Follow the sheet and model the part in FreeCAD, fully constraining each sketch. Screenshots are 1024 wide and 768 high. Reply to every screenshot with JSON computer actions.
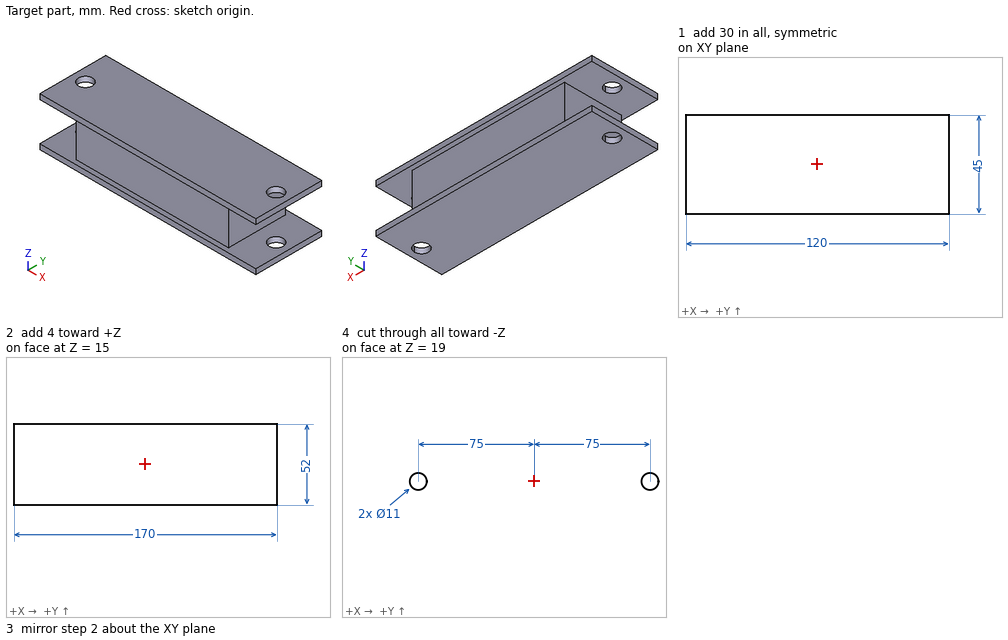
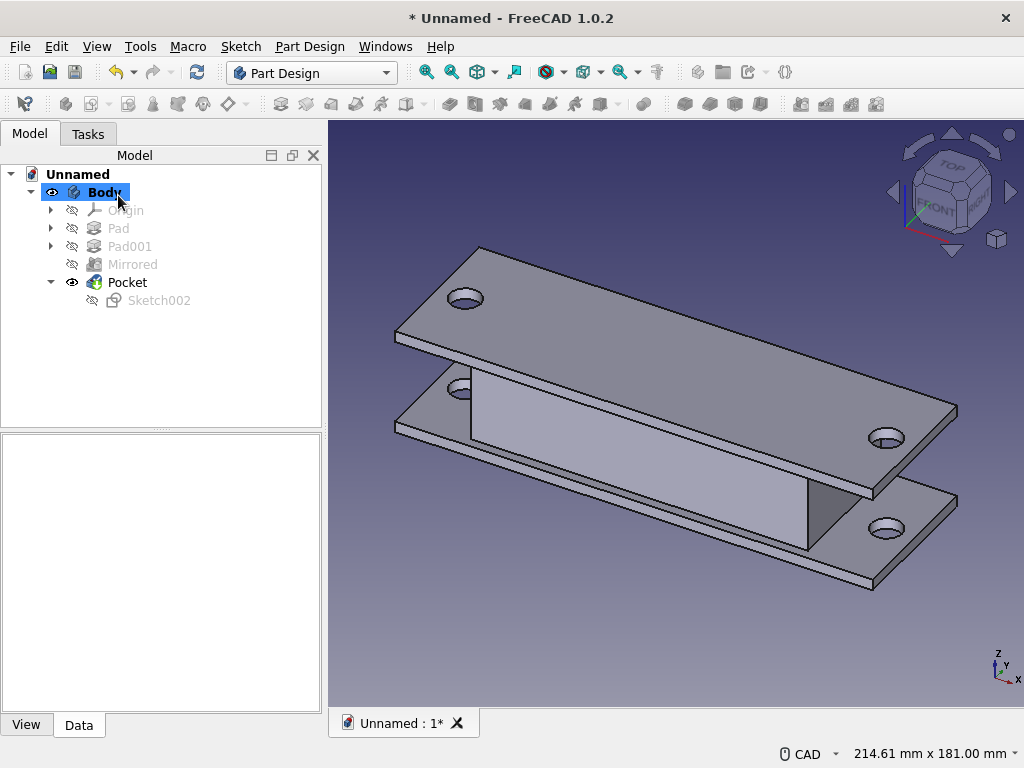
{"action": "key", "text": "0"}